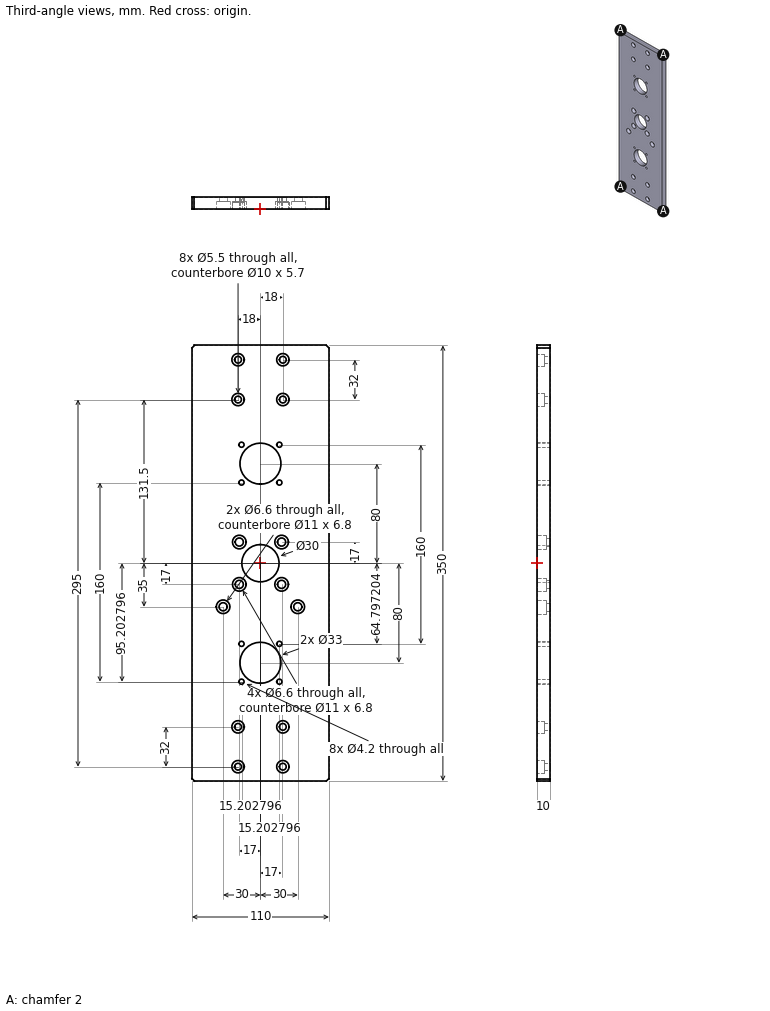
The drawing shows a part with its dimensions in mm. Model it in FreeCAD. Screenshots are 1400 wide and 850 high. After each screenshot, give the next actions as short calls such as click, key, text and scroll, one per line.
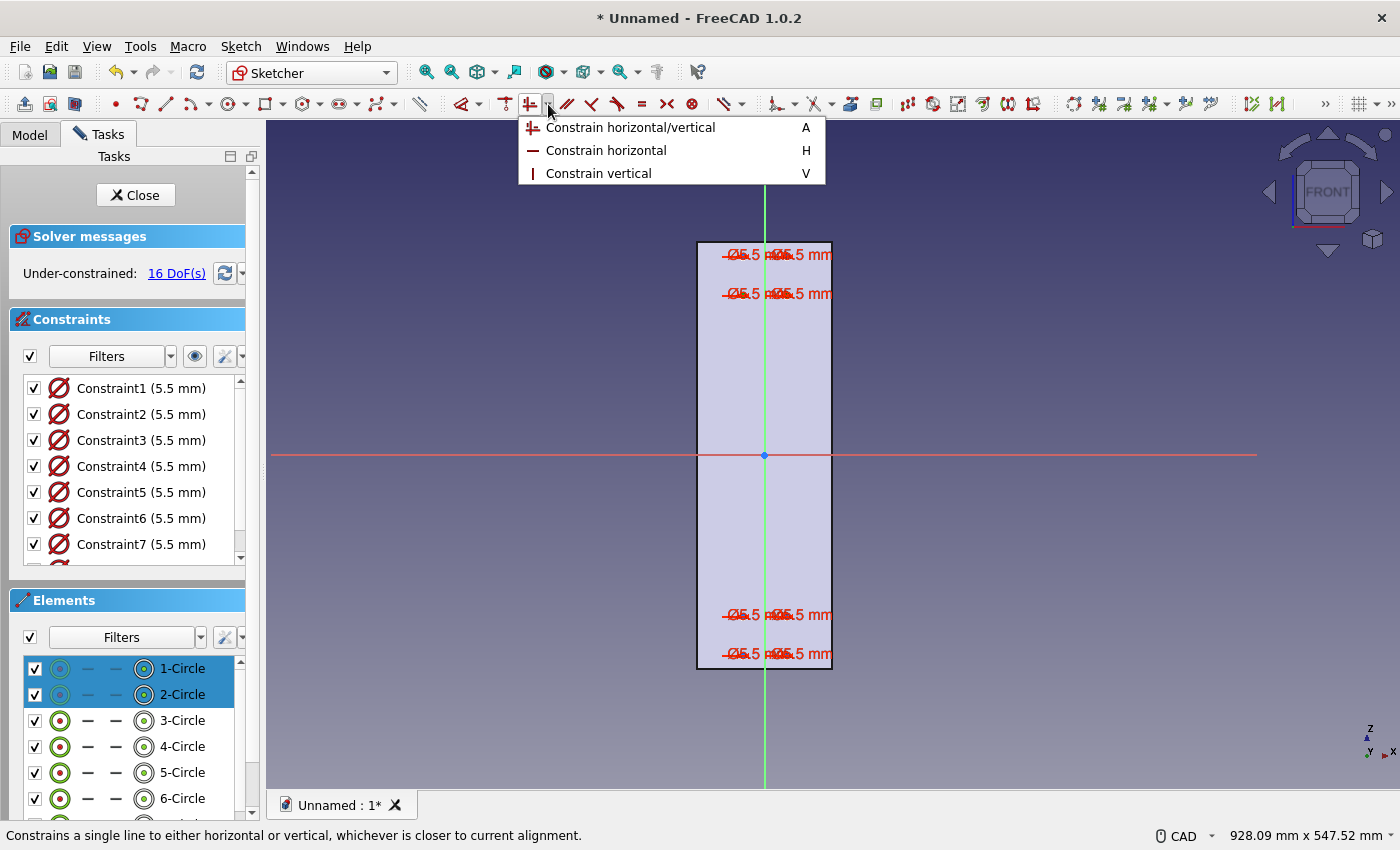
click(672, 150)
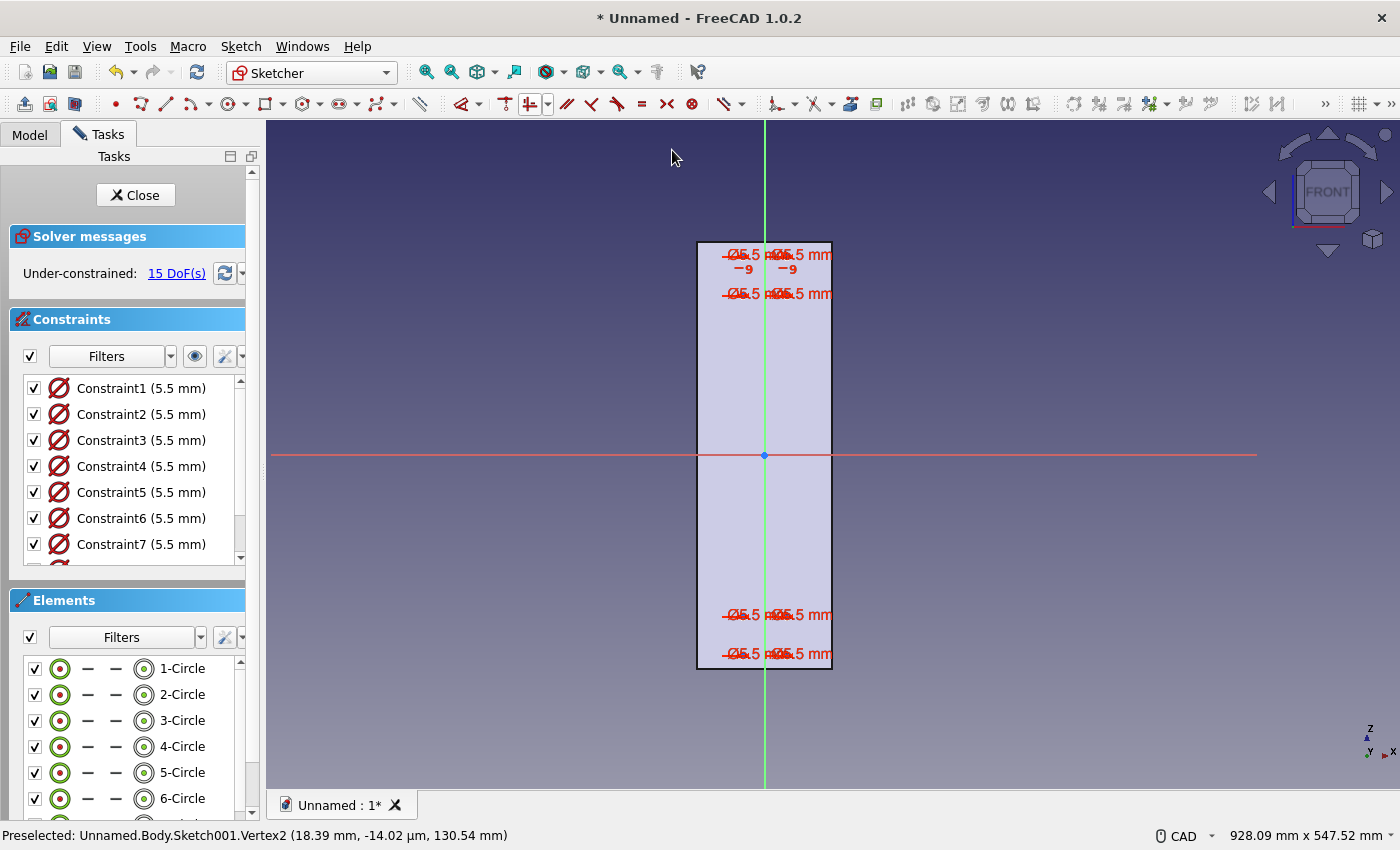
click(787, 296)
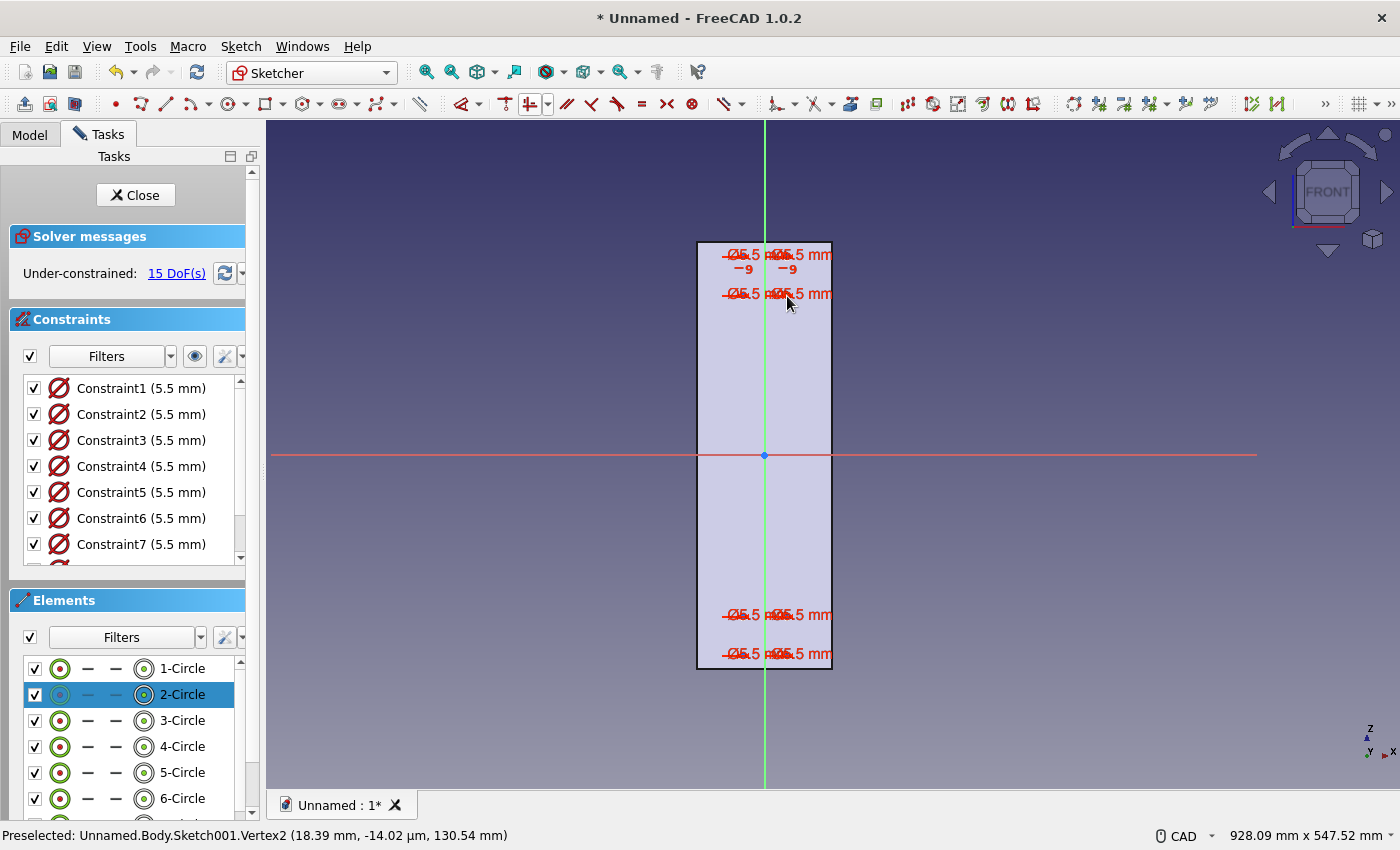
click(787, 257)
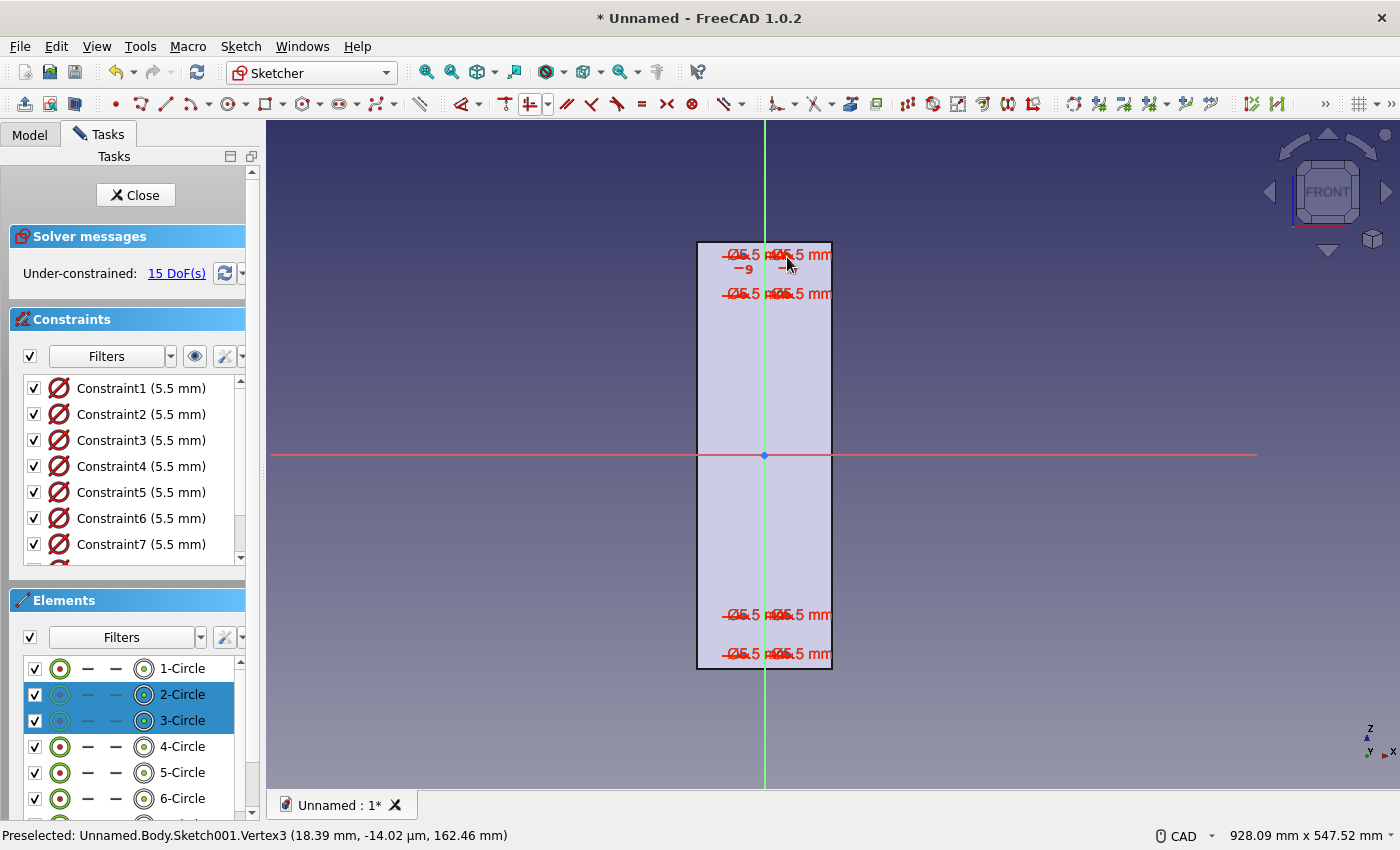
key(v)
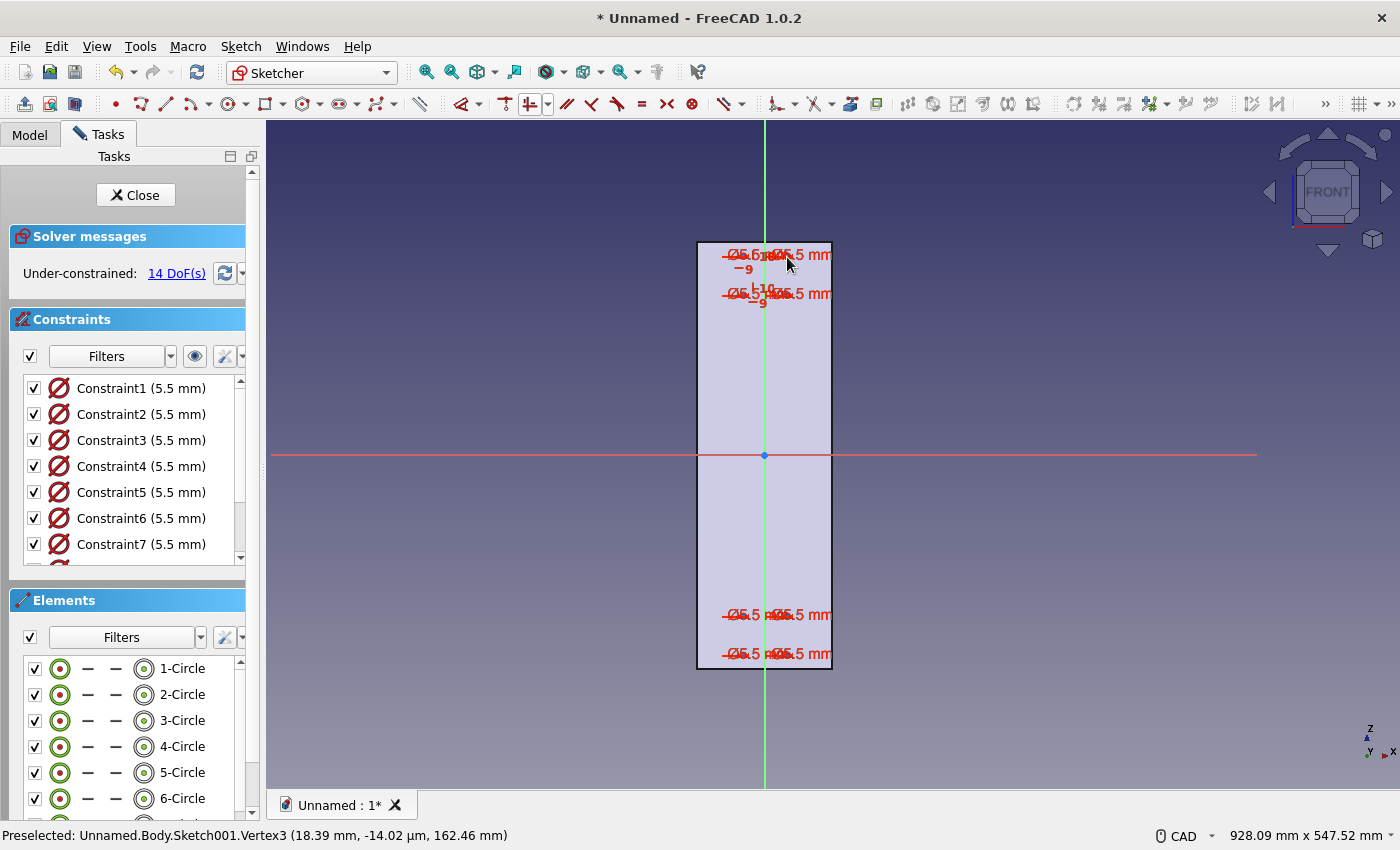
click(743, 296)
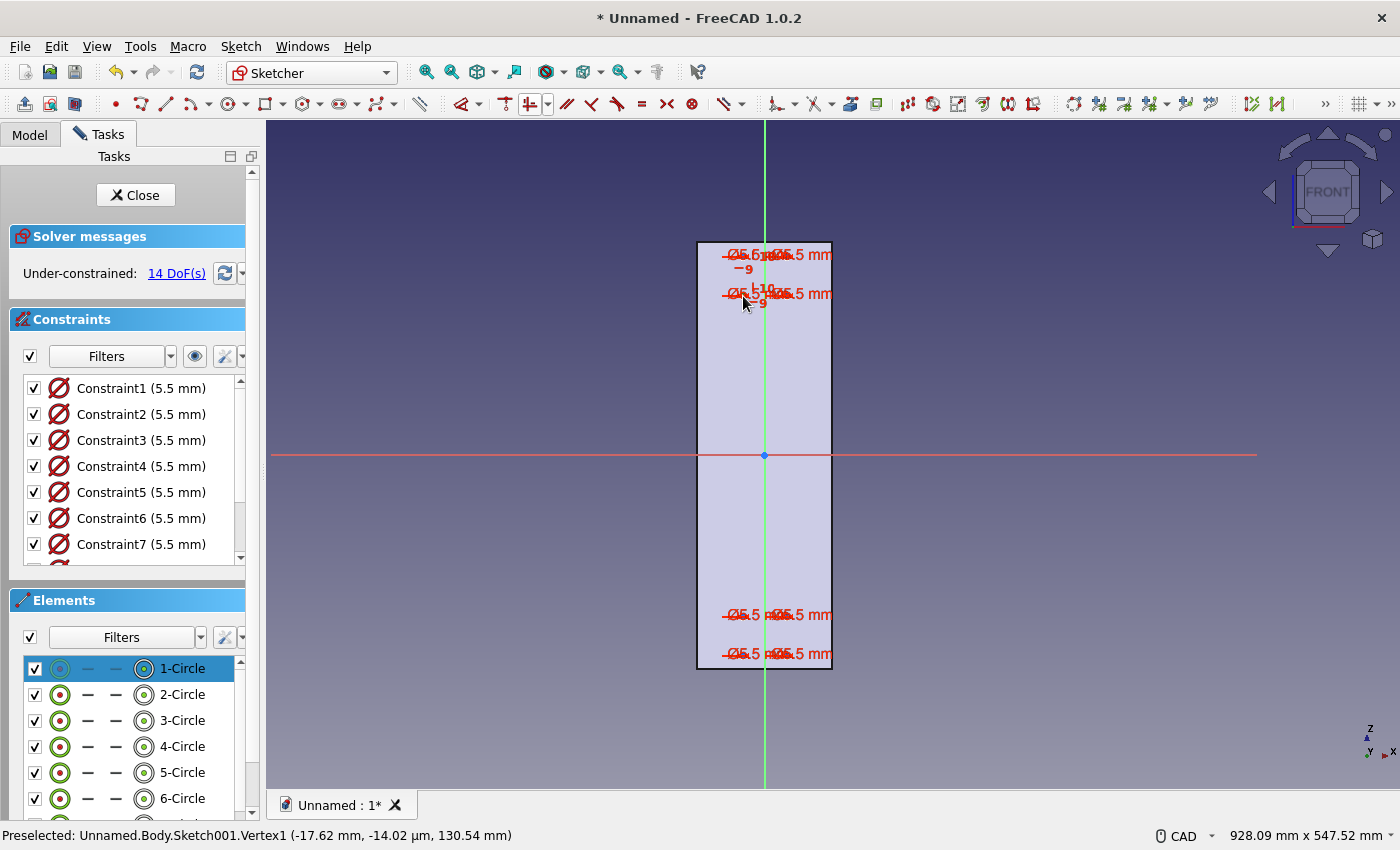
click(743, 257)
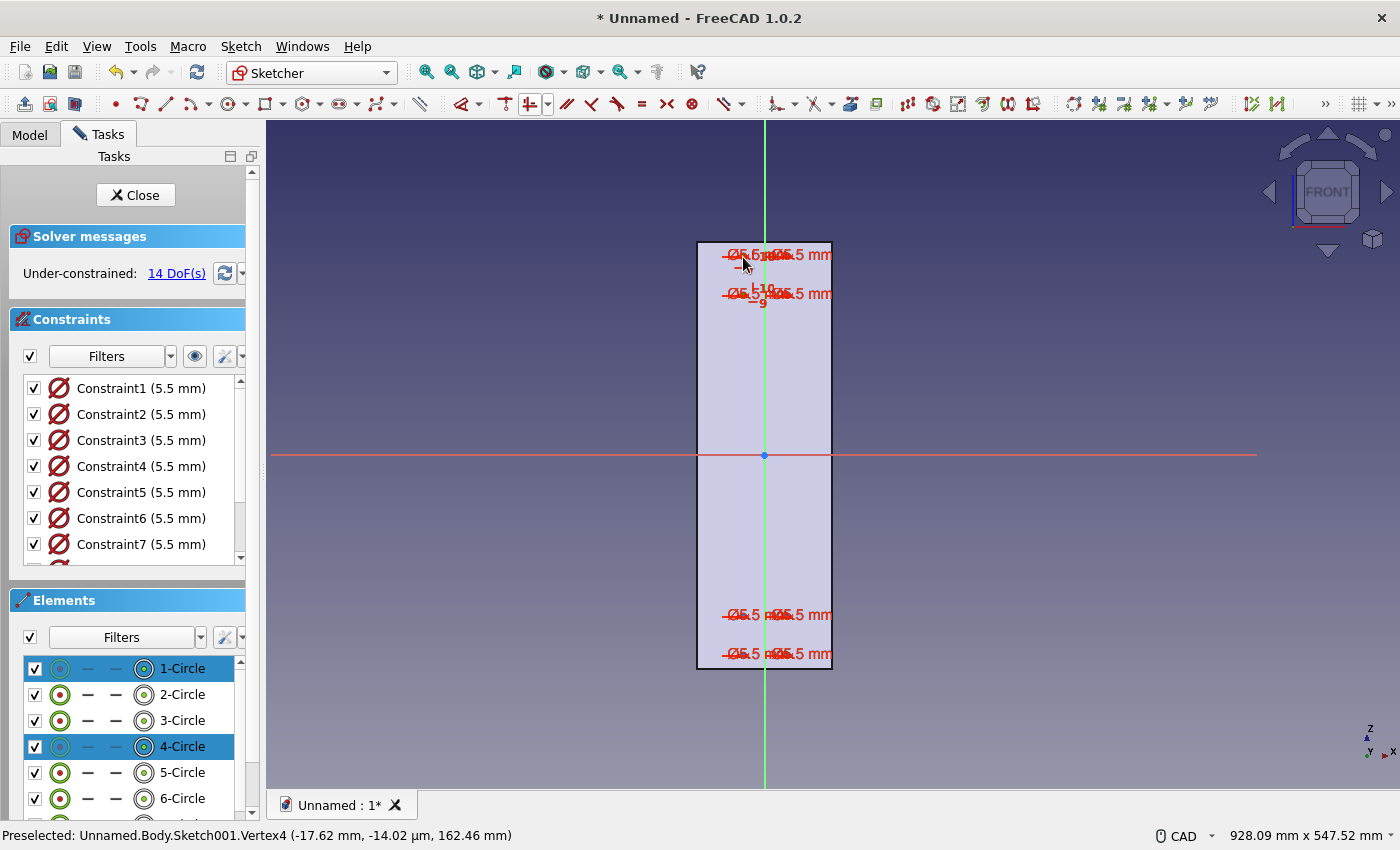
key(v)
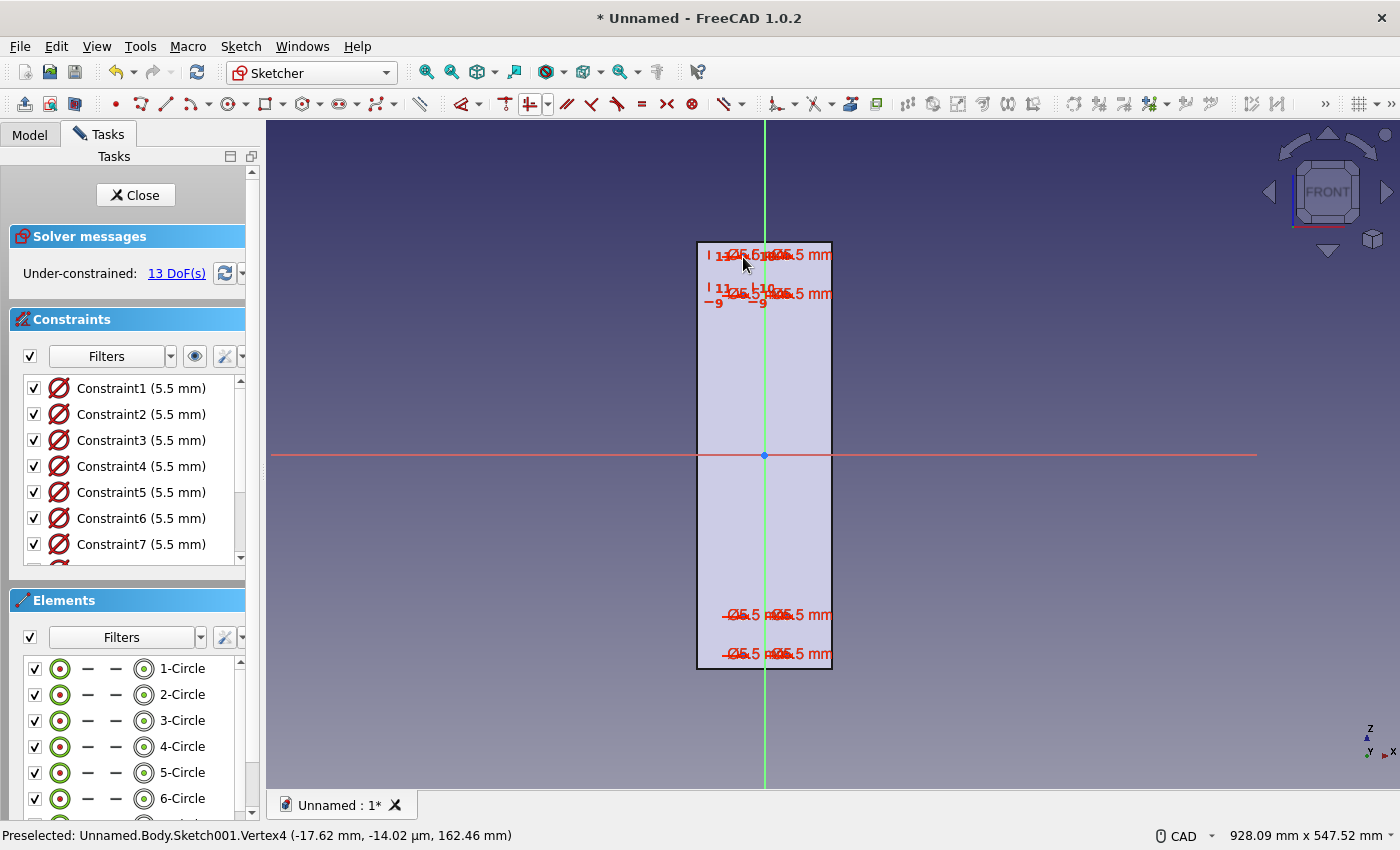
click(787, 257)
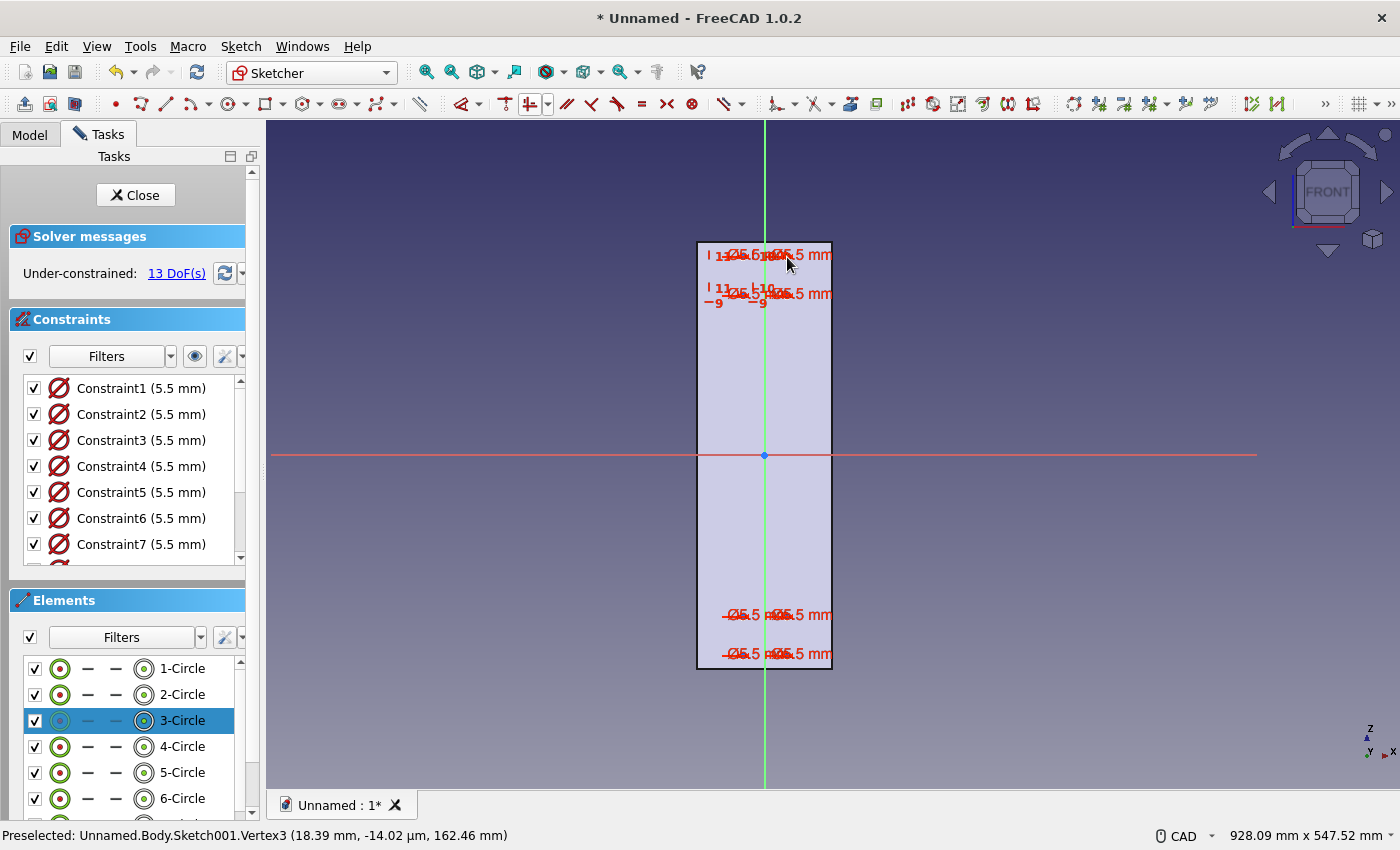
click(743, 257)